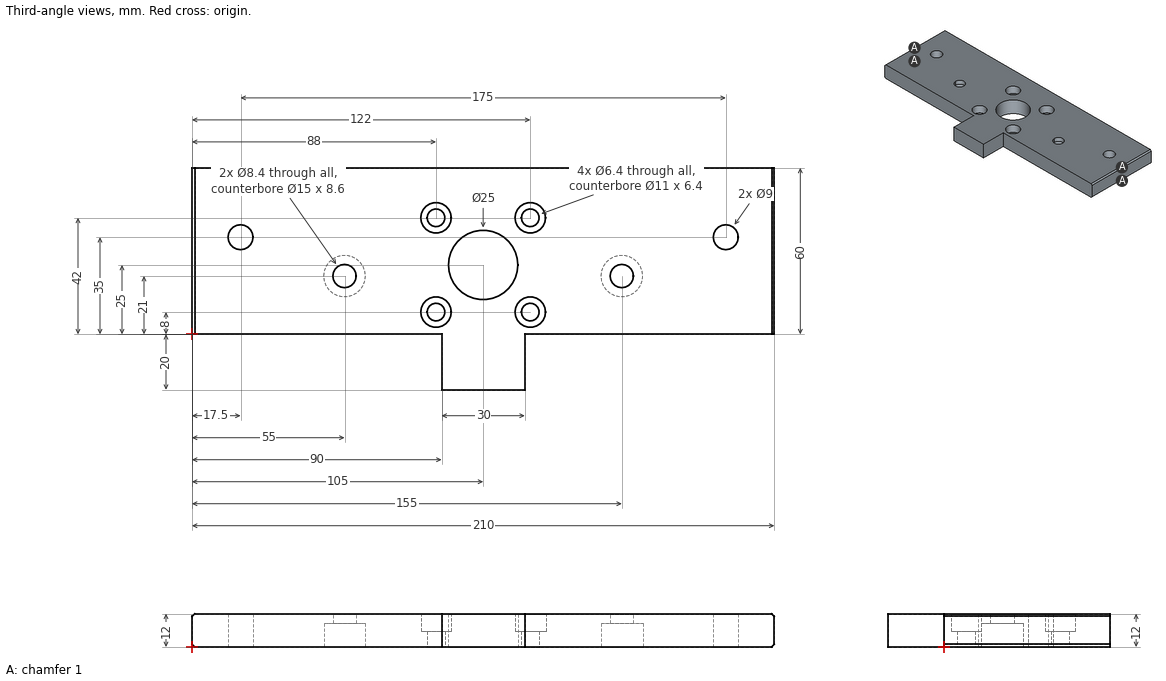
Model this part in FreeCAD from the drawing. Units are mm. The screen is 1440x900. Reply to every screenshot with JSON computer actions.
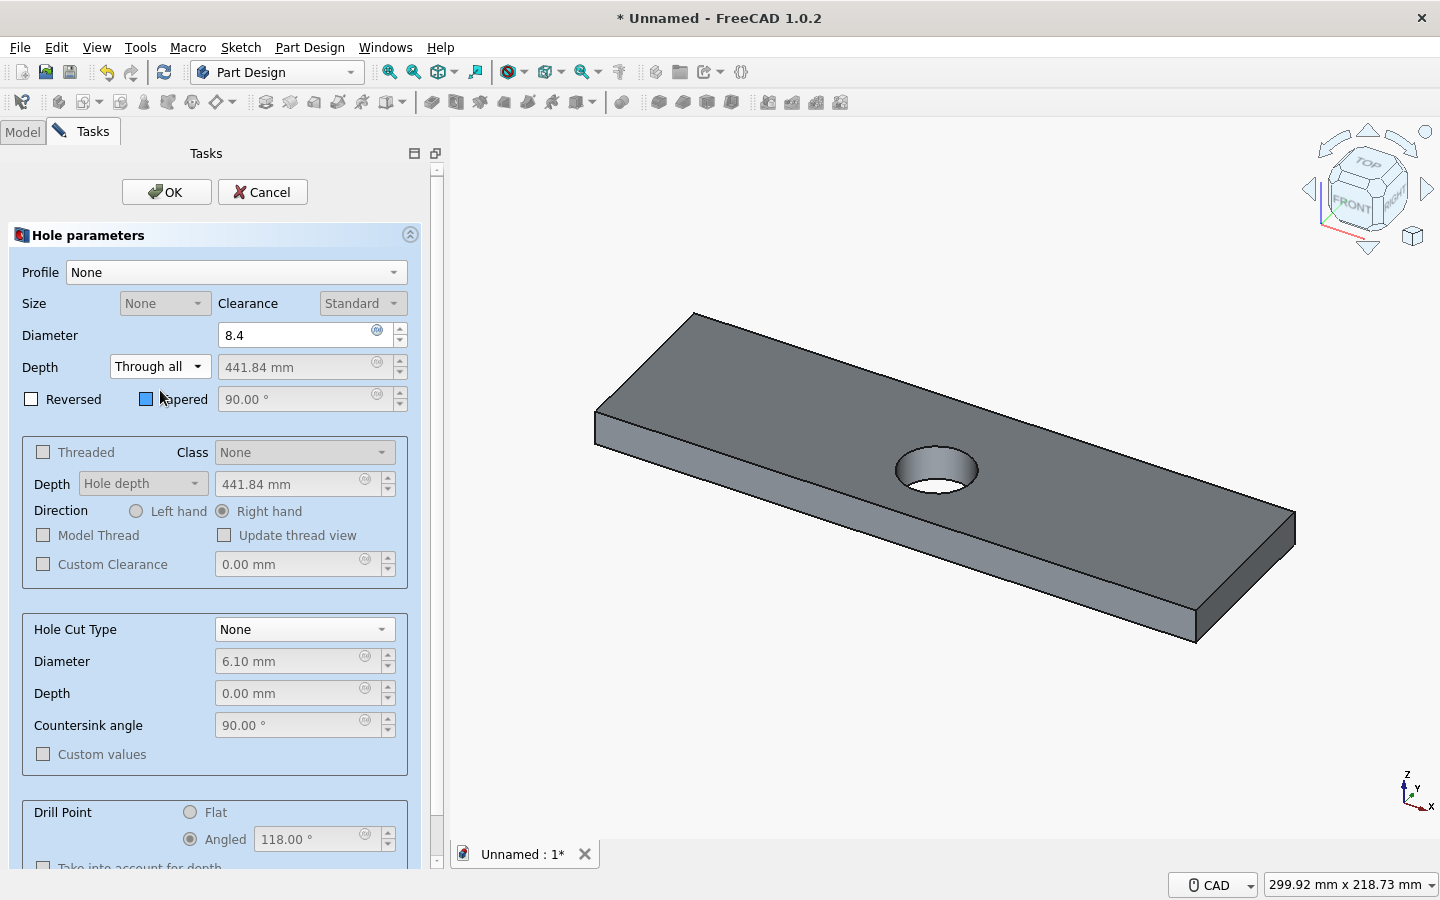
{"action": "left_click", "coordinate": [30, 399]}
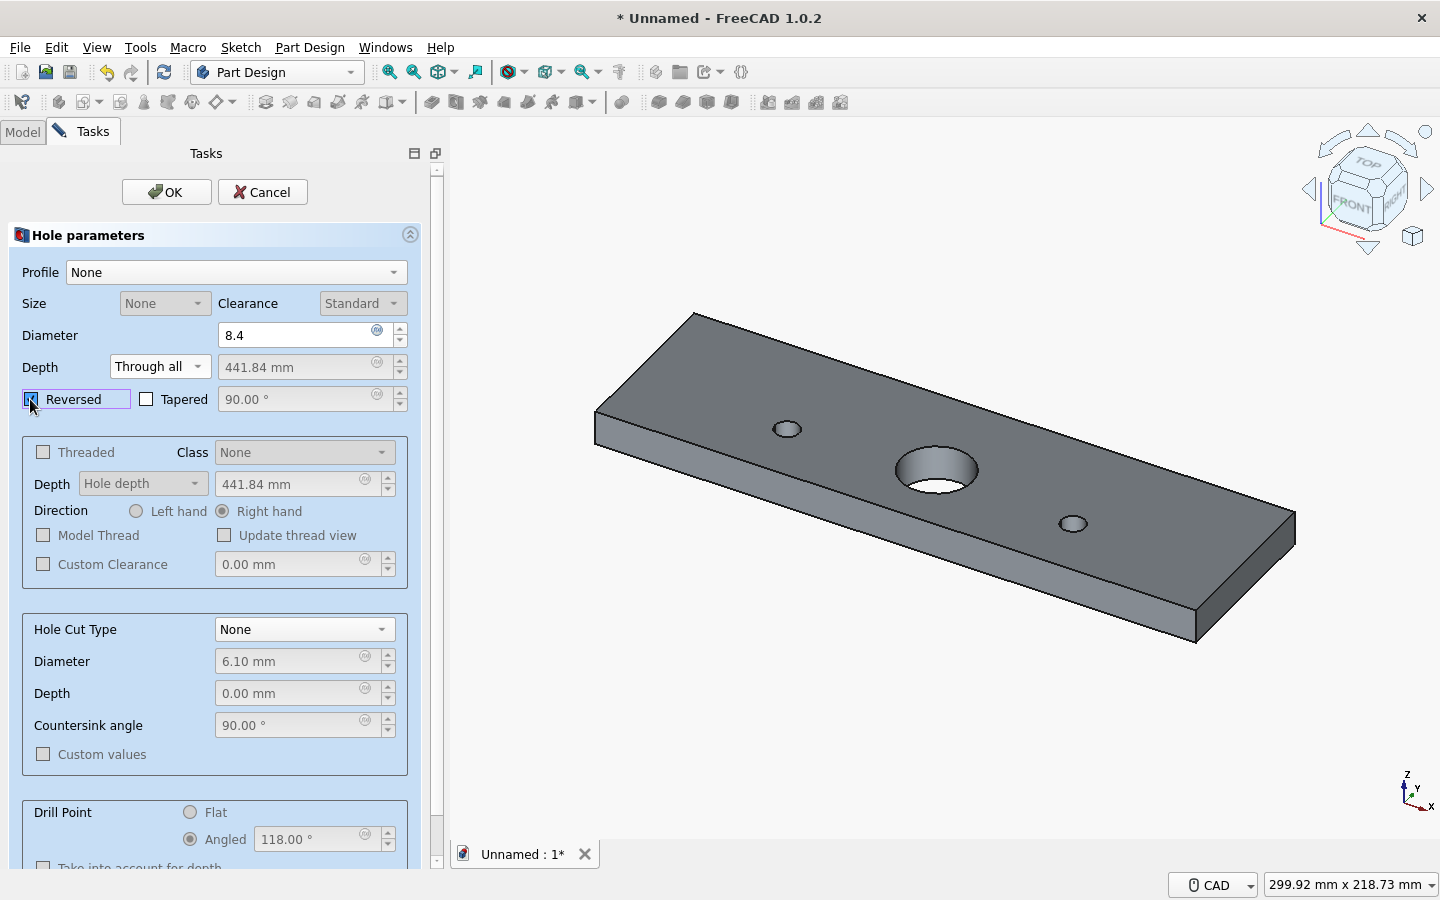
{"action": "left_click", "coordinate": [306, 630]}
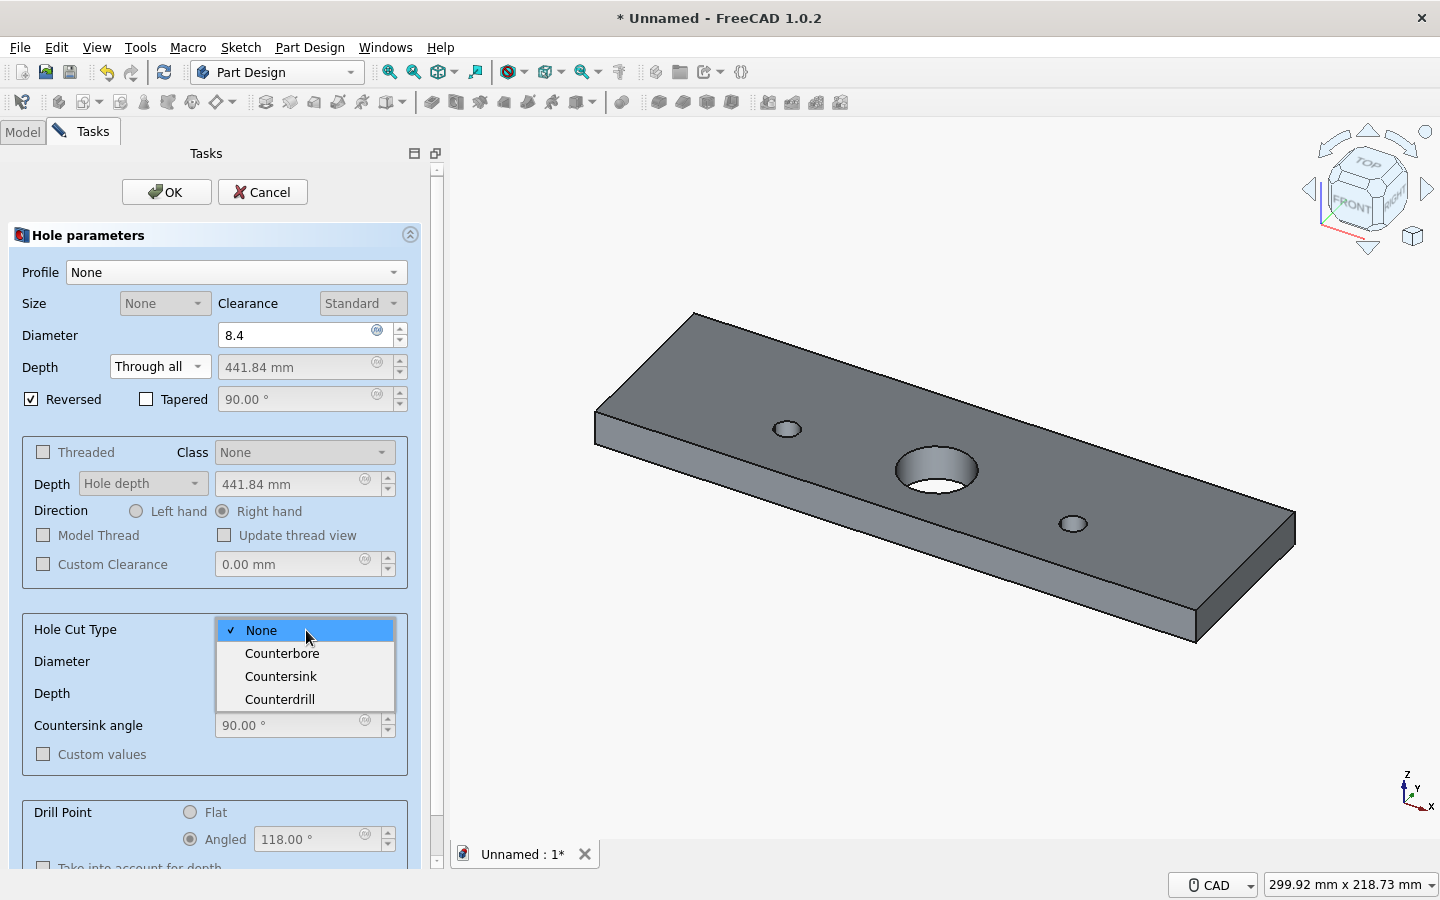
{"action": "left_click", "coordinate": [304, 654]}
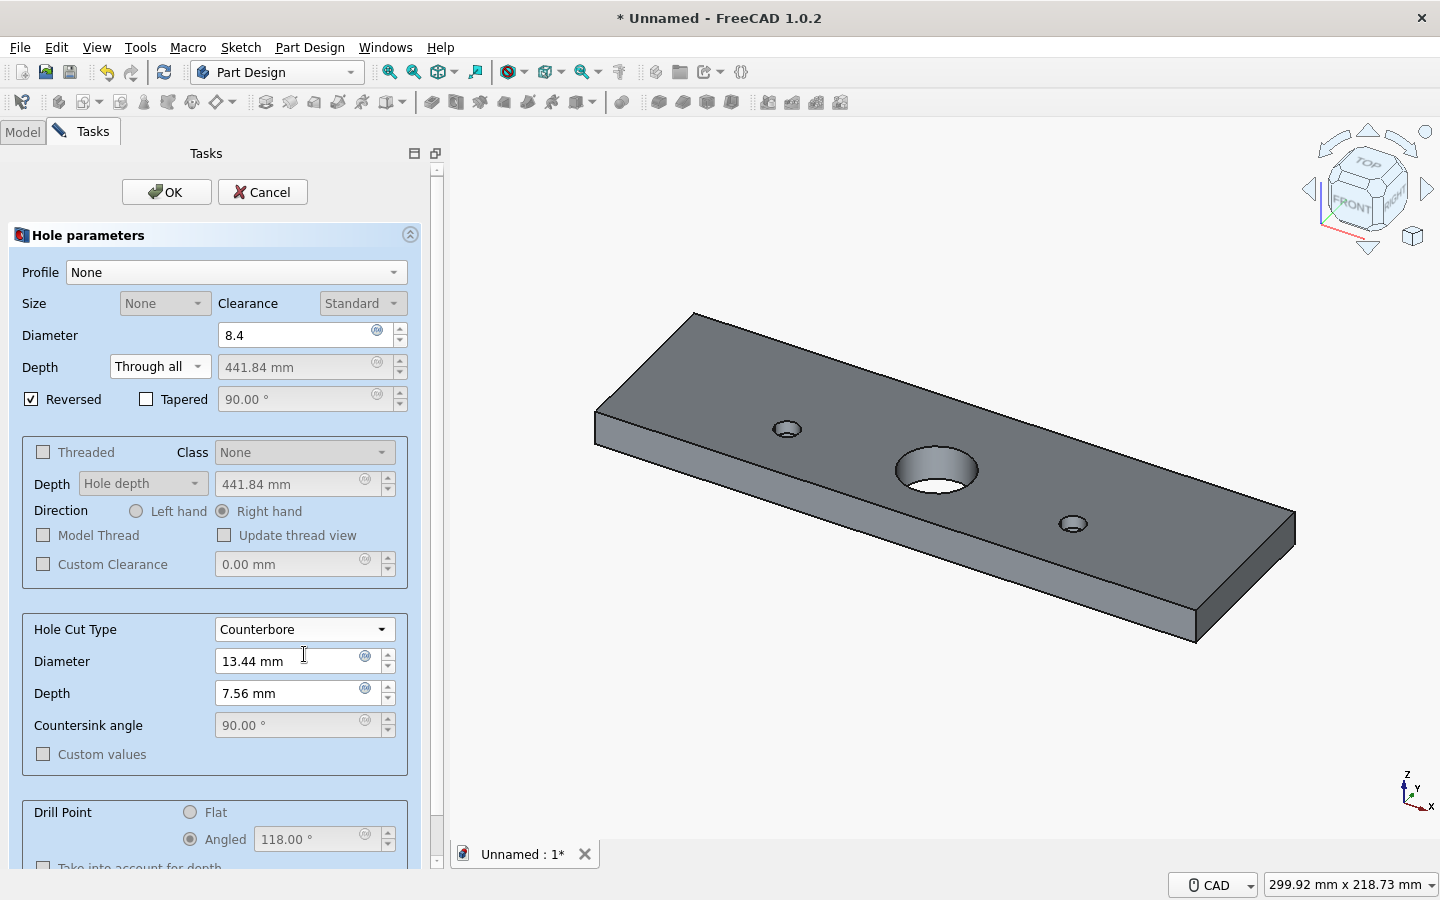
{"action": "triple_click", "coordinate": [298, 661]}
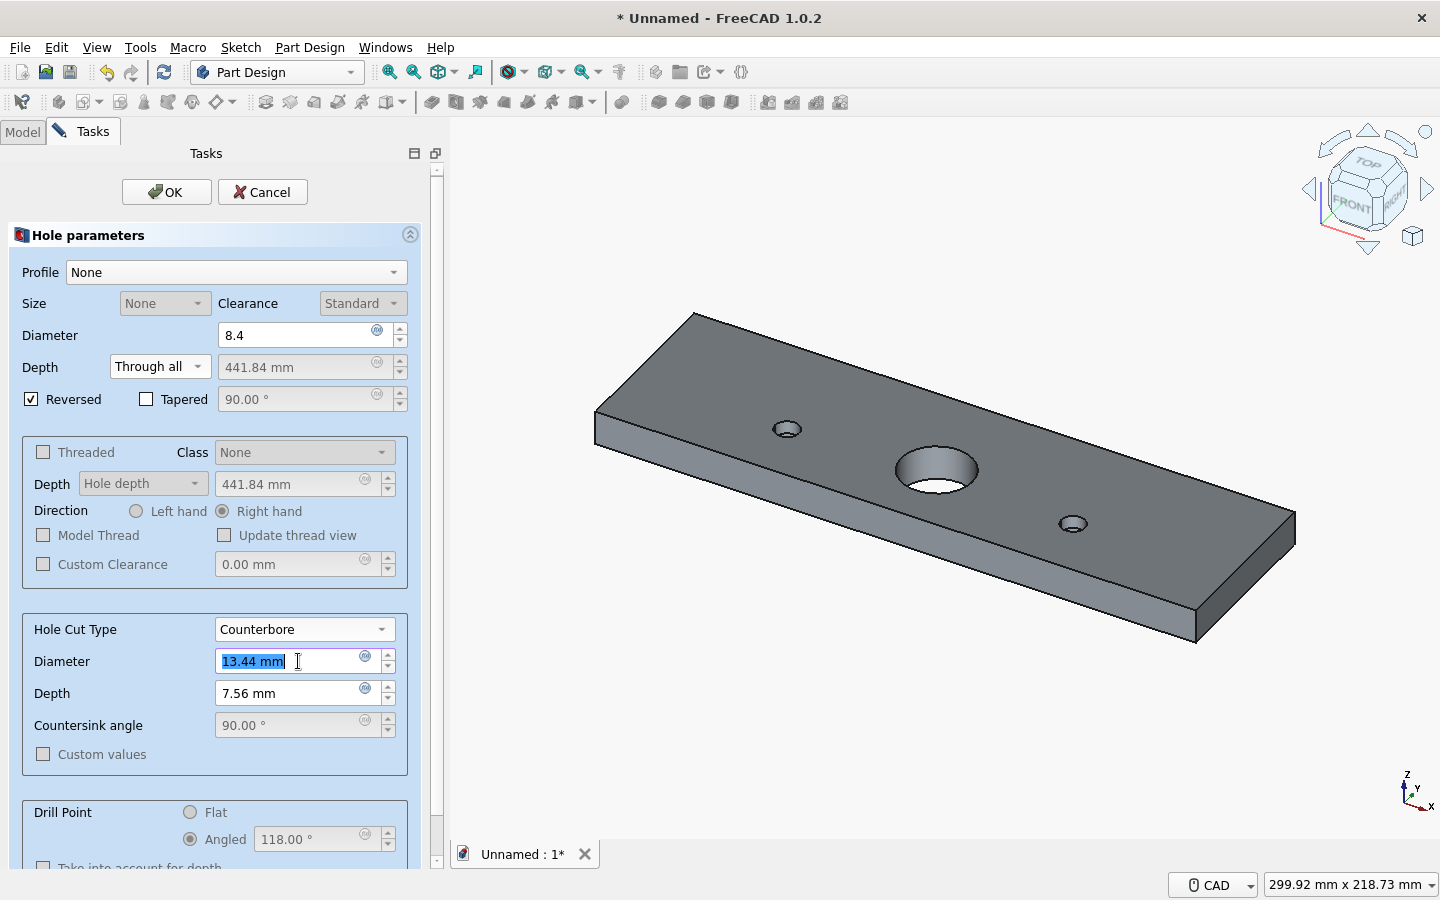
{"action": "type", "text": "15"}
{"action": "key", "text": "Tab"}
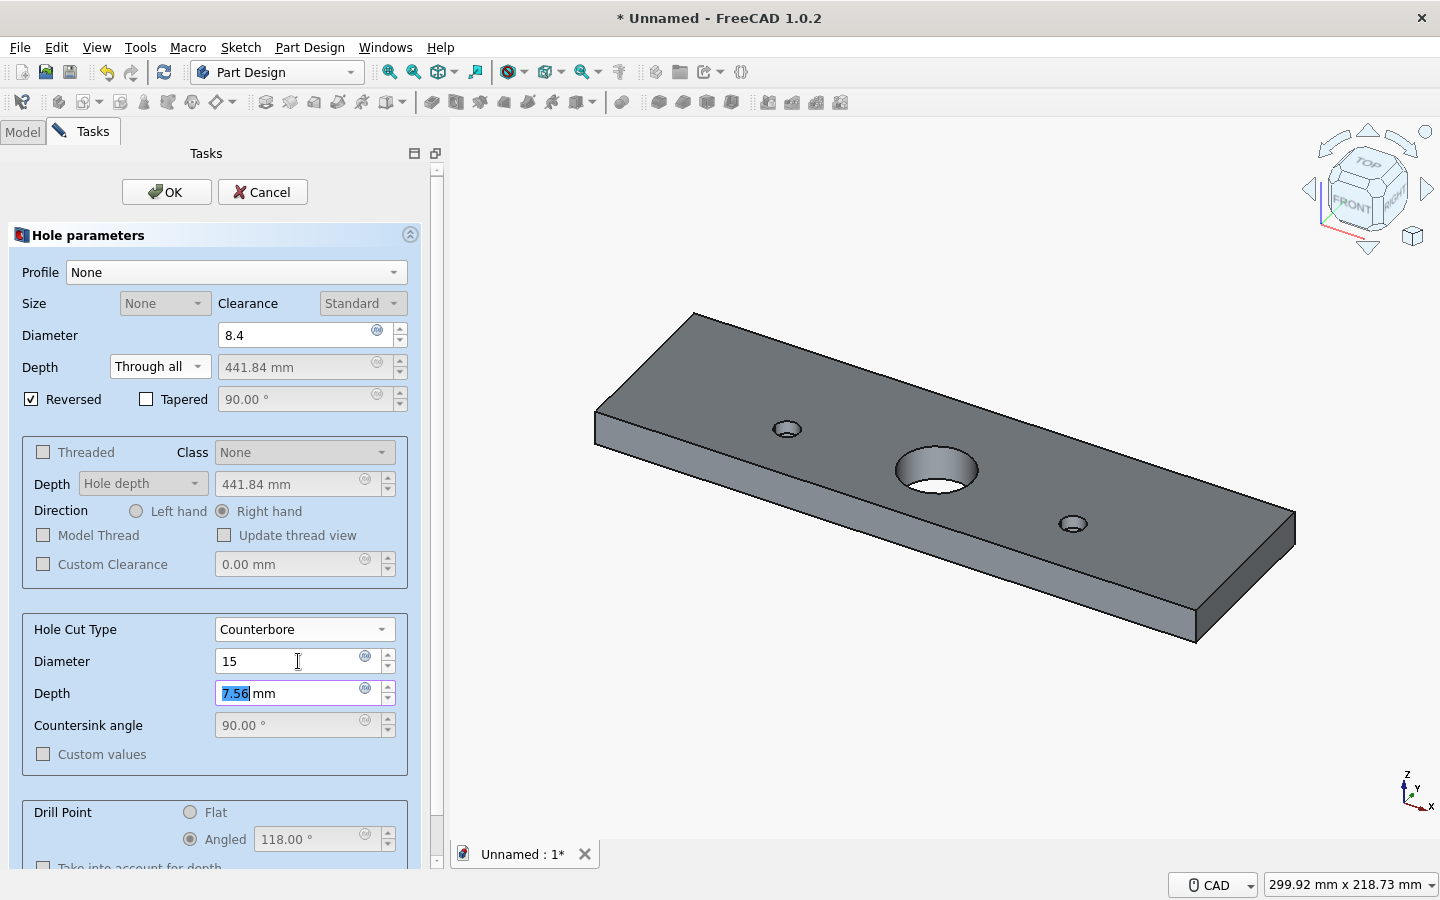
{"action": "type", "text": "8.6"}
{"action": "key", "text": "Tab"}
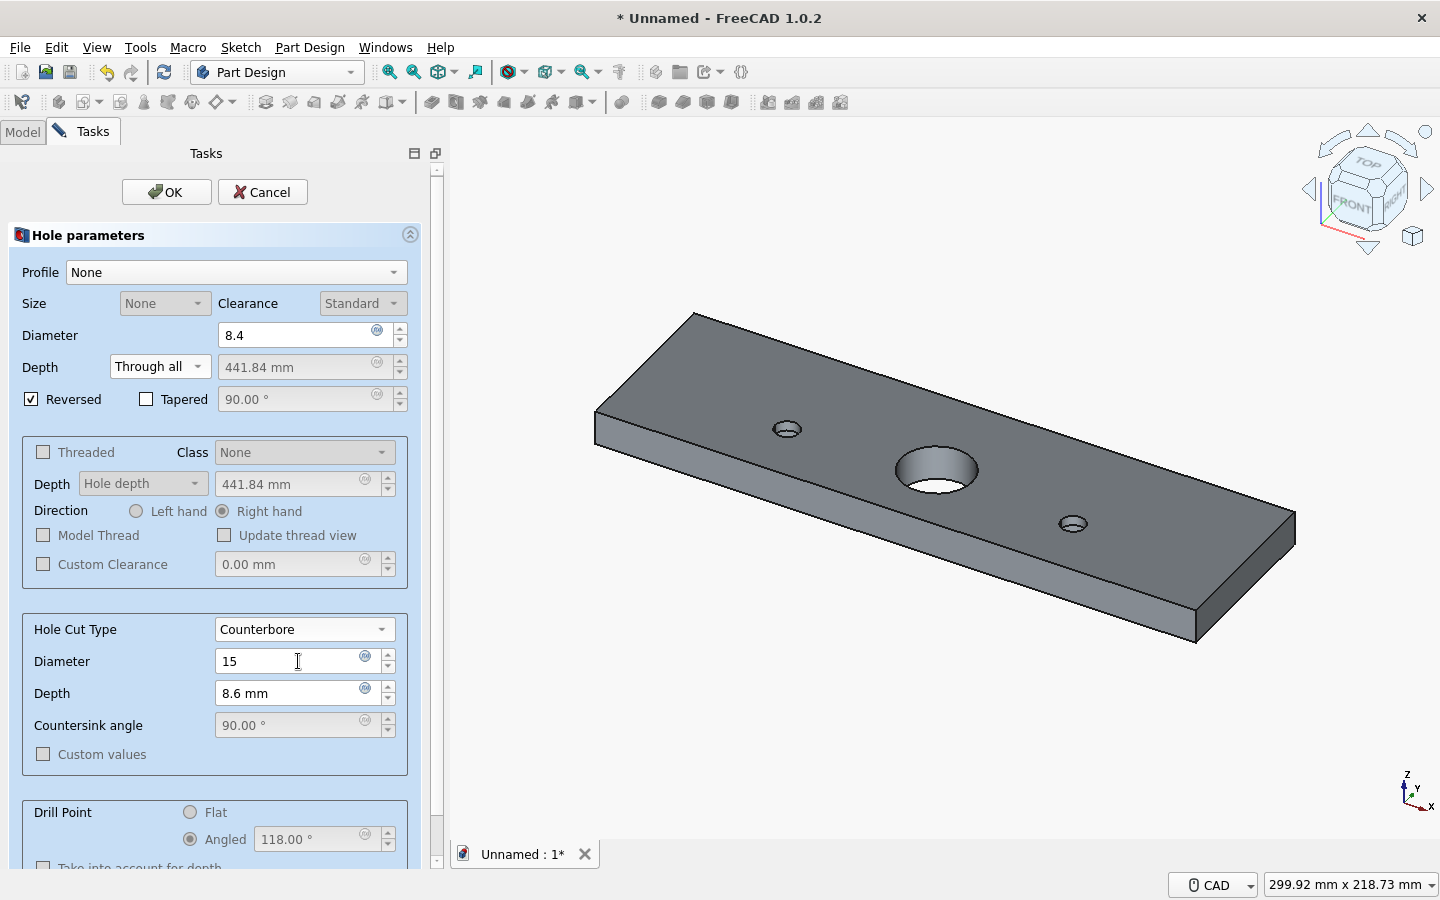
{"action": "left_click", "coordinate": [167, 192]}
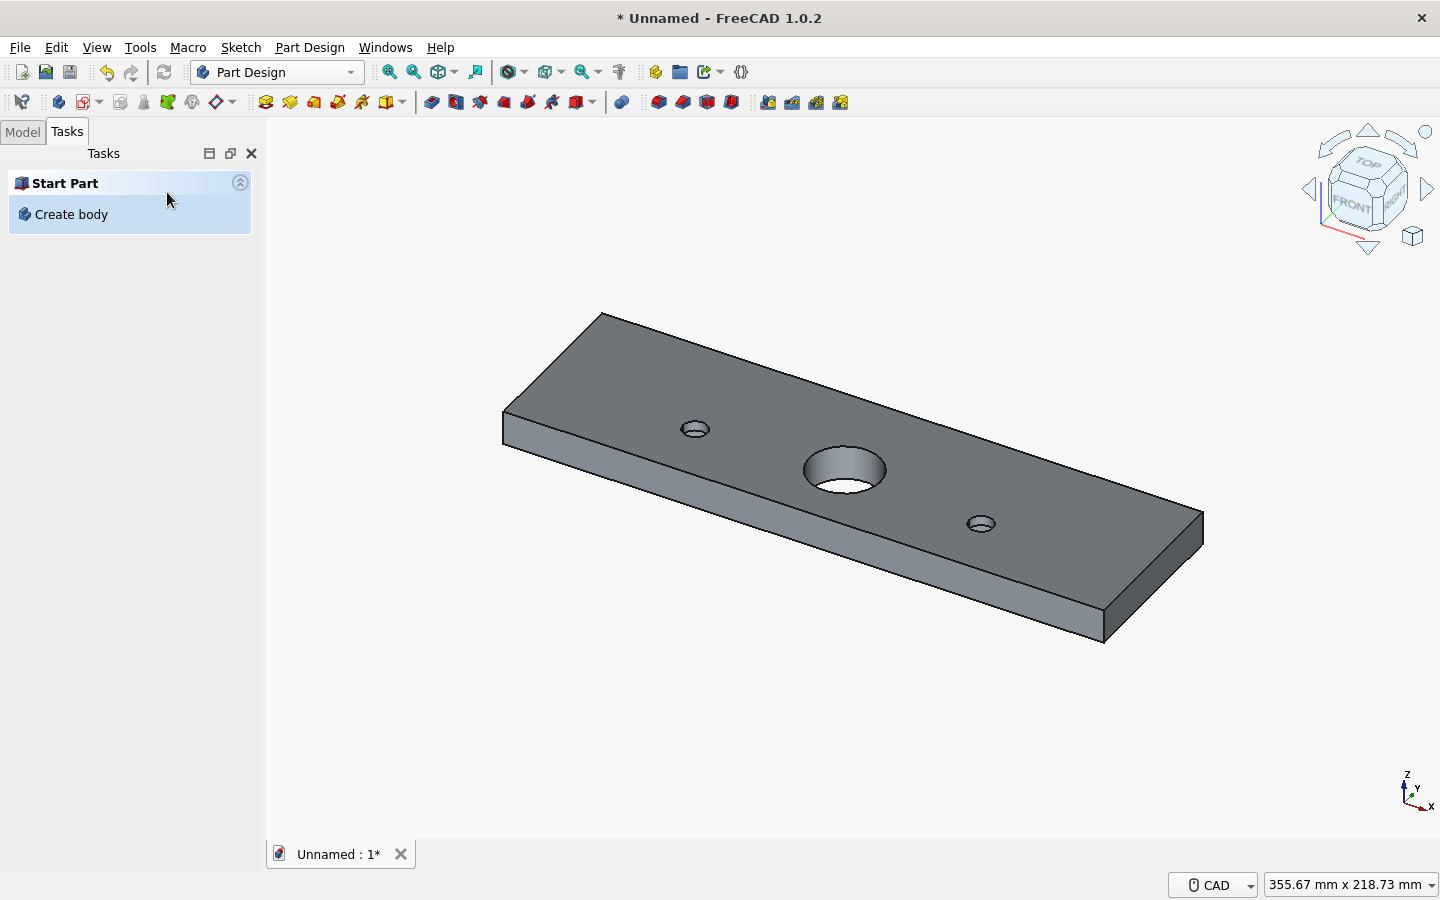
{"action": "left_click", "coordinate": [953, 475]}